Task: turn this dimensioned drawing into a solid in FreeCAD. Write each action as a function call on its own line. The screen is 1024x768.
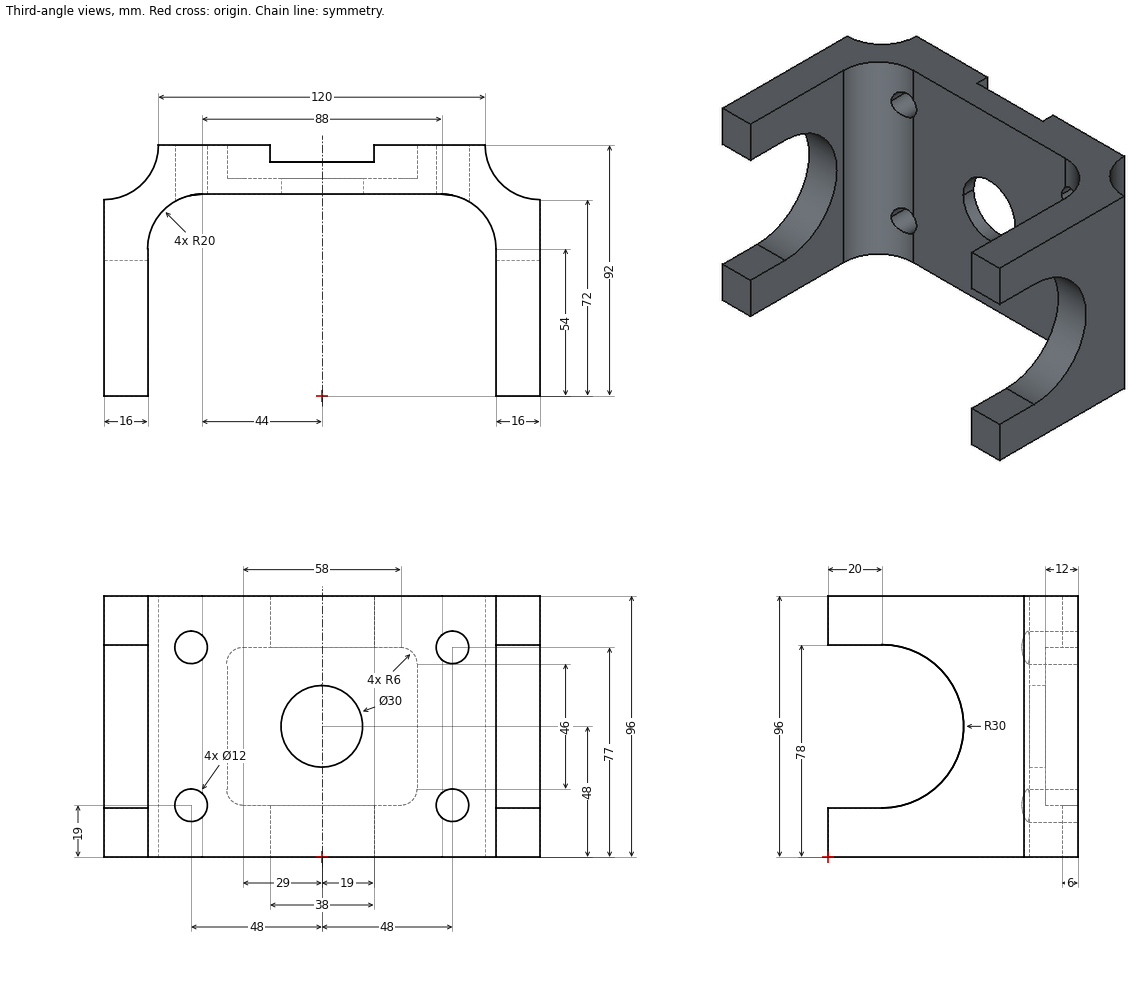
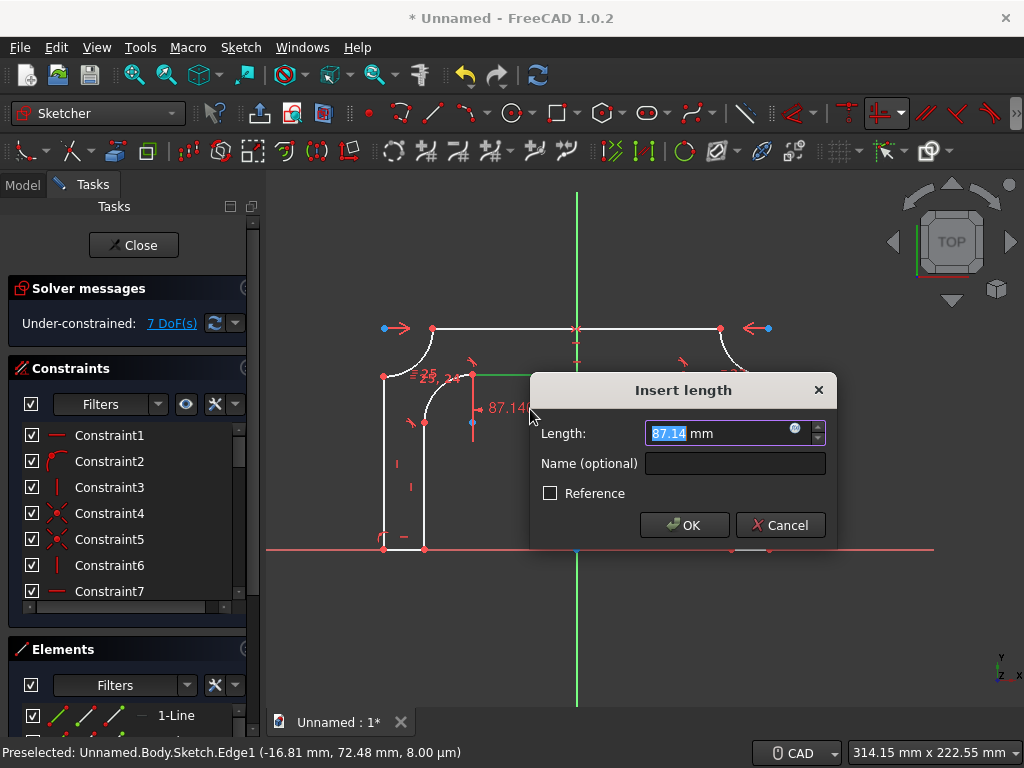
text(88)
key(Return)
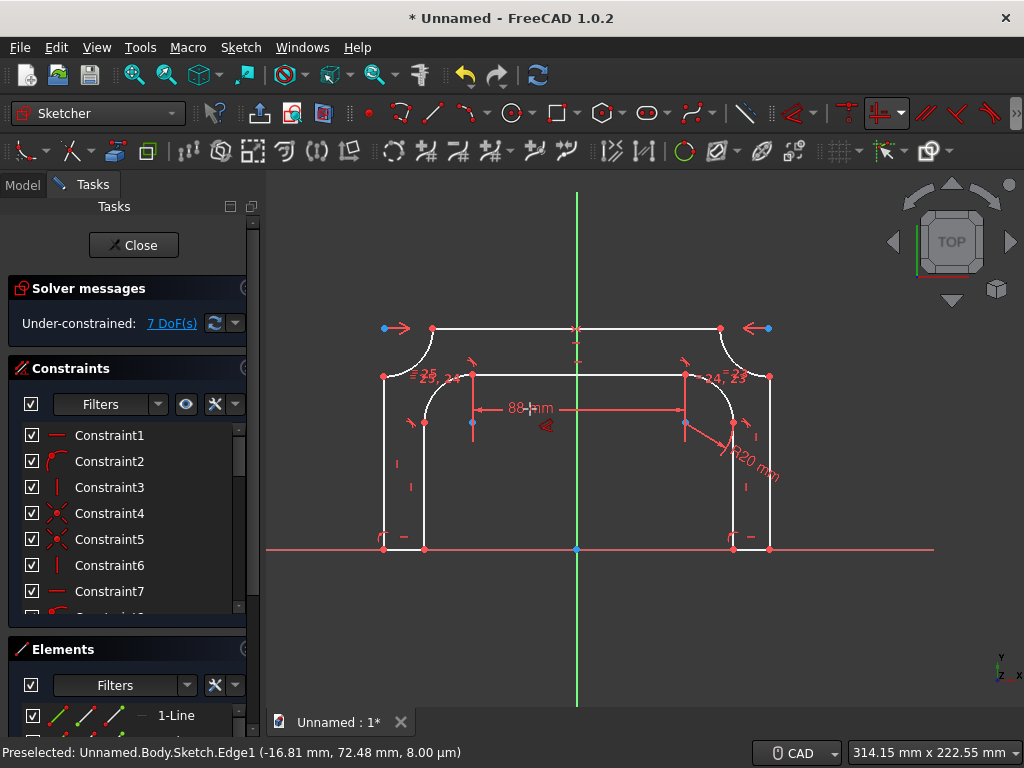
click(733, 461)
click(699, 486)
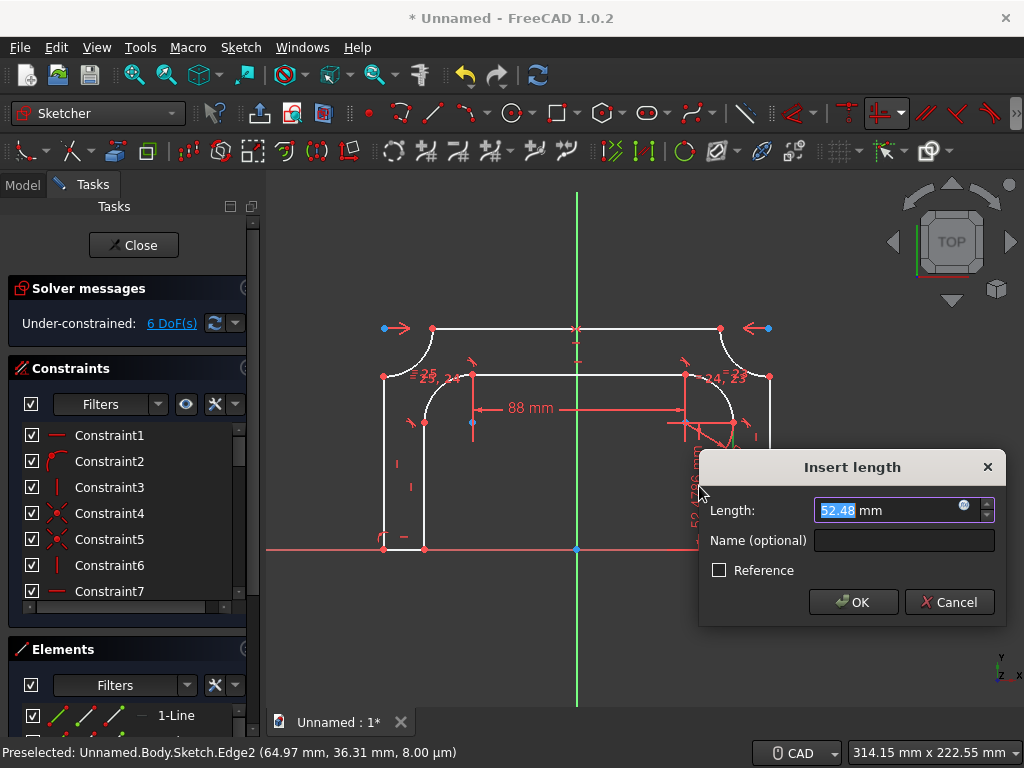
text(54)
key(Return)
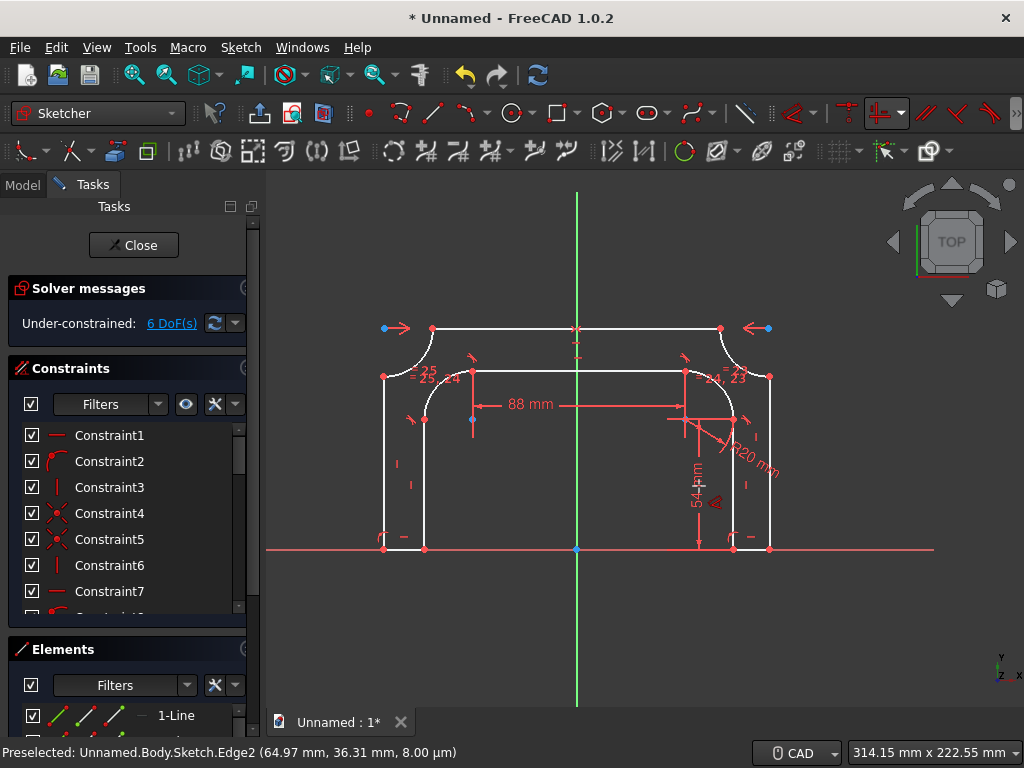
scroll(744, 550, up, 2)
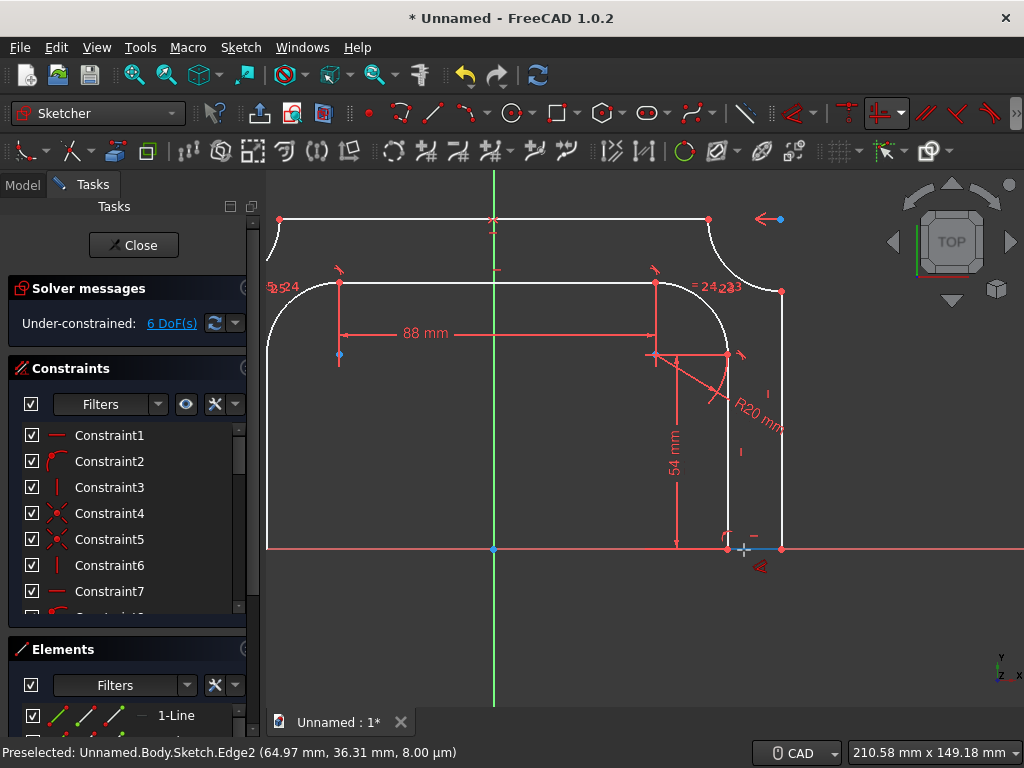
click(744, 549)
click(755, 583)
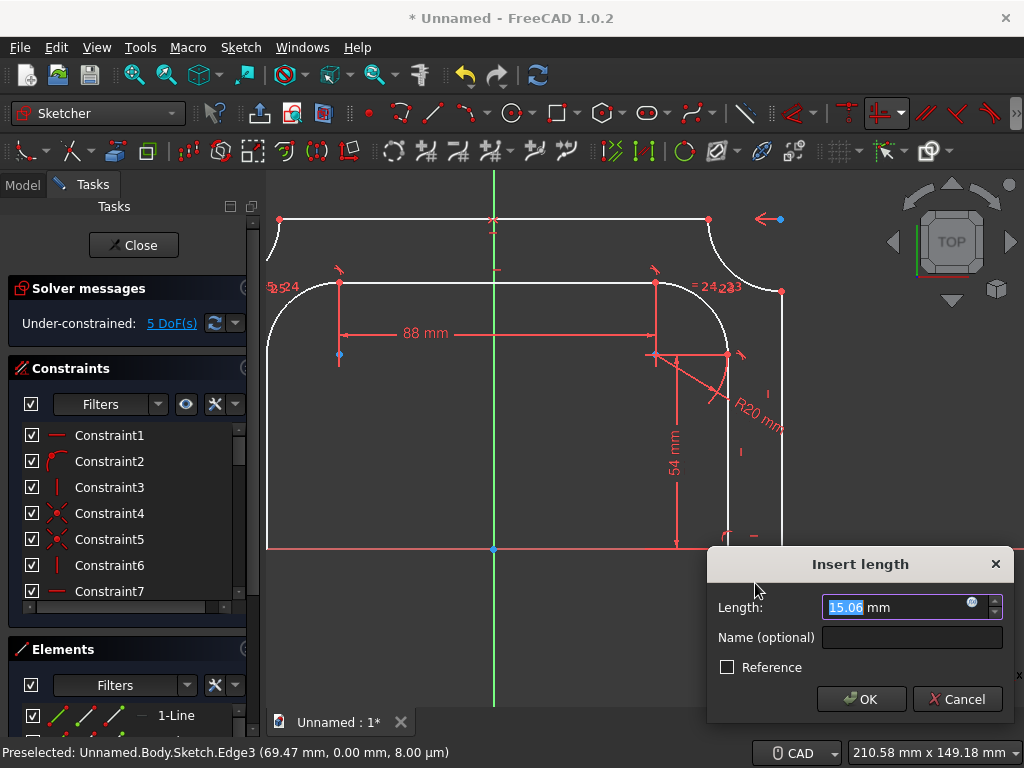
text(16)
key(Return)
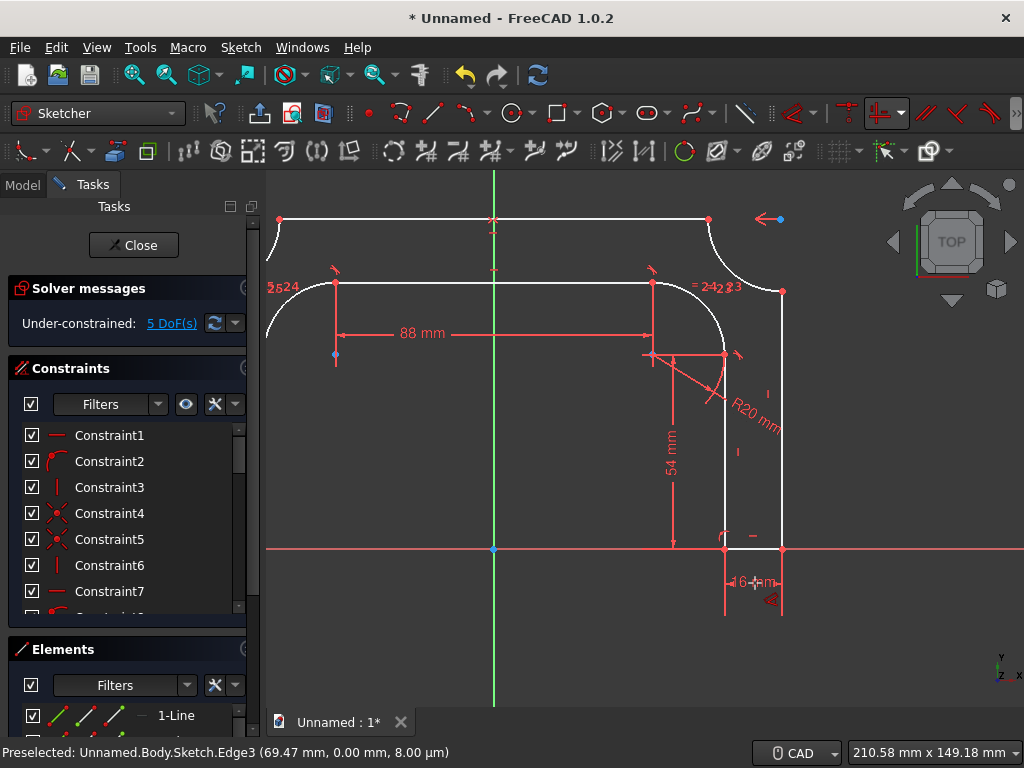
click(782, 472)
click(816, 361)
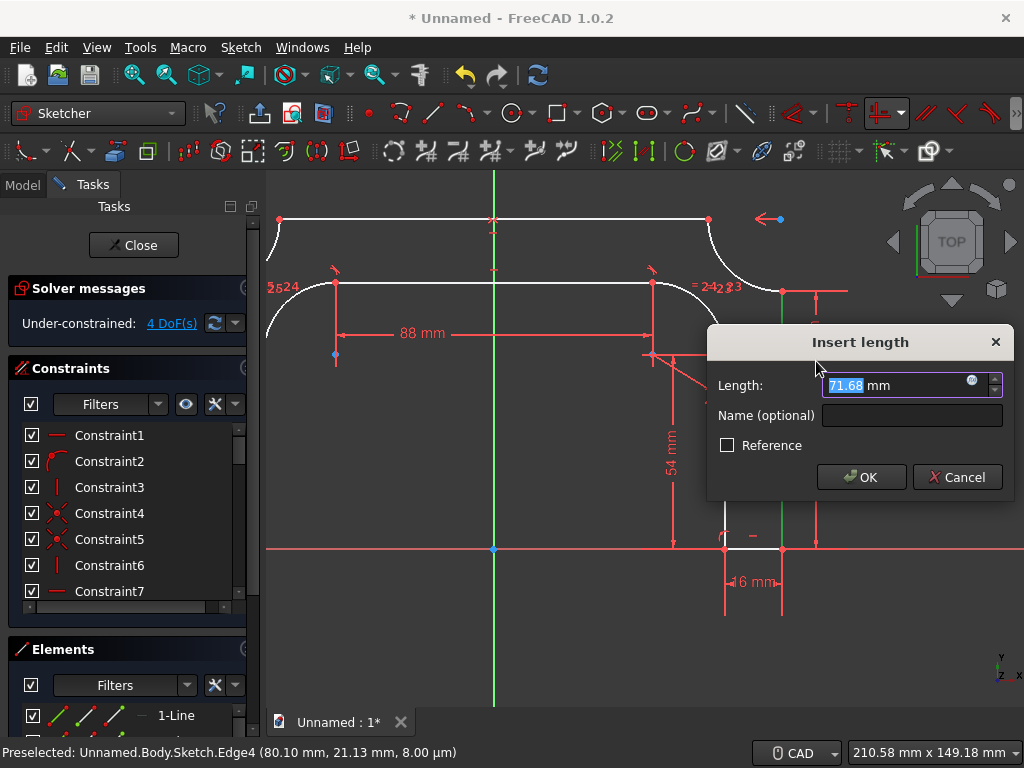
text(72)
key(Return)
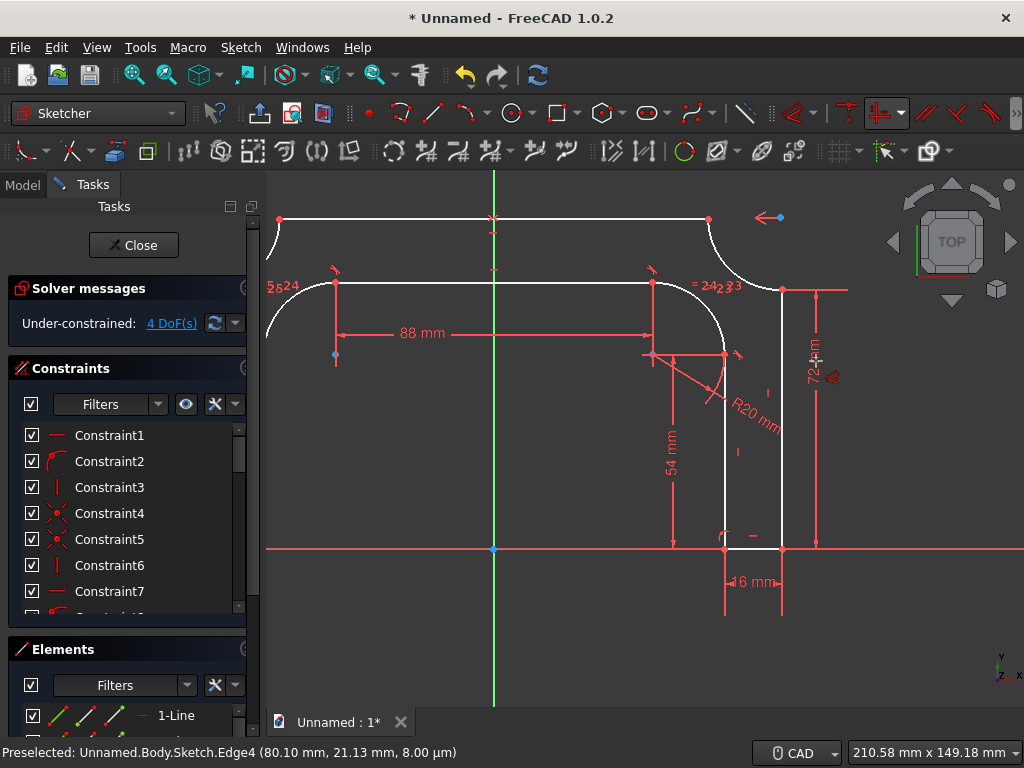
scroll(744, 550, down, 2)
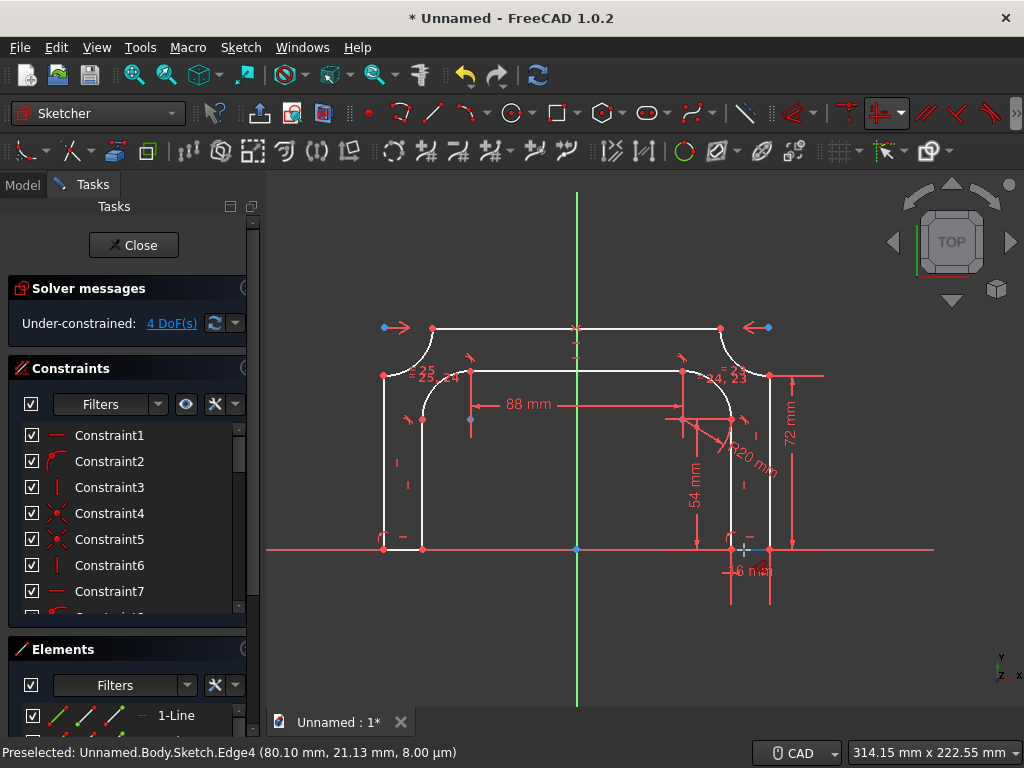
click(395, 550)
click(403, 584)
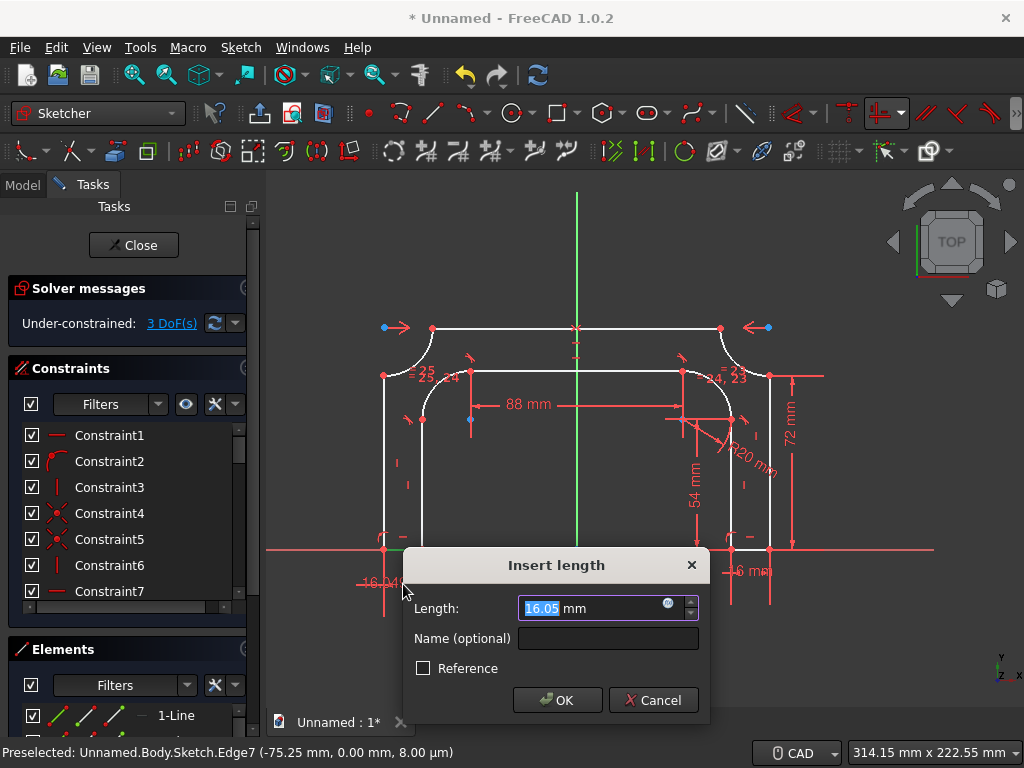
text(16)
key(Return)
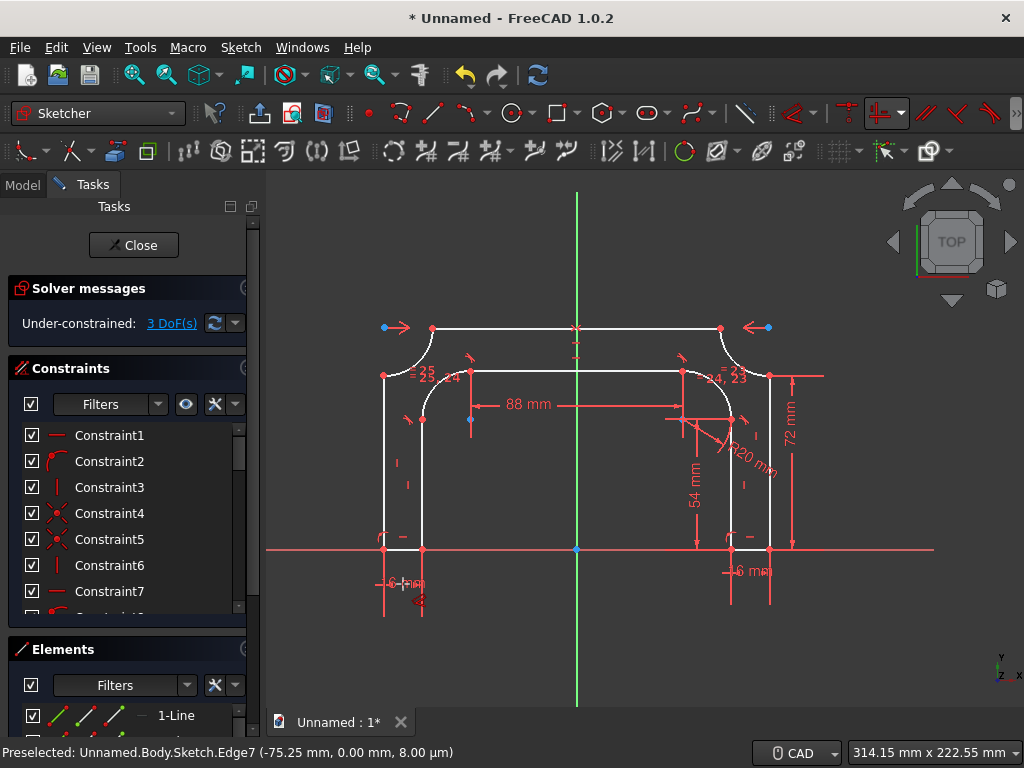
click(634, 329)
click(511, 295)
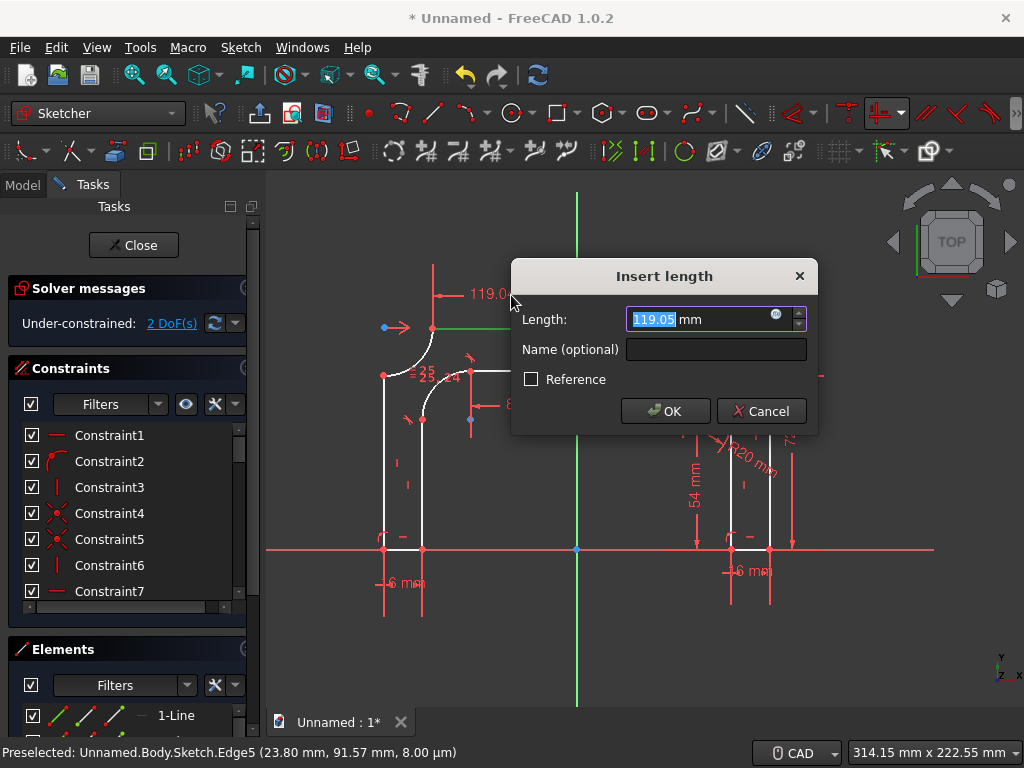
text(120)
key(Return)